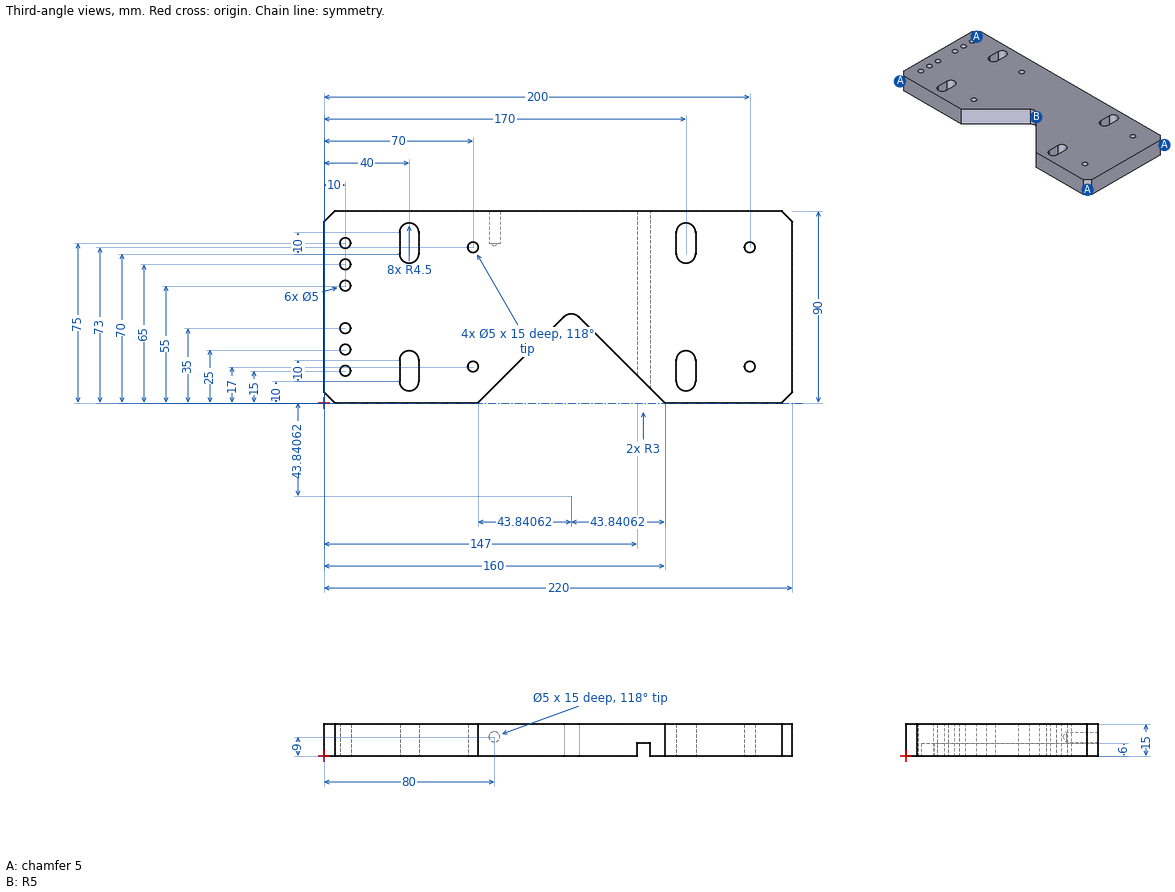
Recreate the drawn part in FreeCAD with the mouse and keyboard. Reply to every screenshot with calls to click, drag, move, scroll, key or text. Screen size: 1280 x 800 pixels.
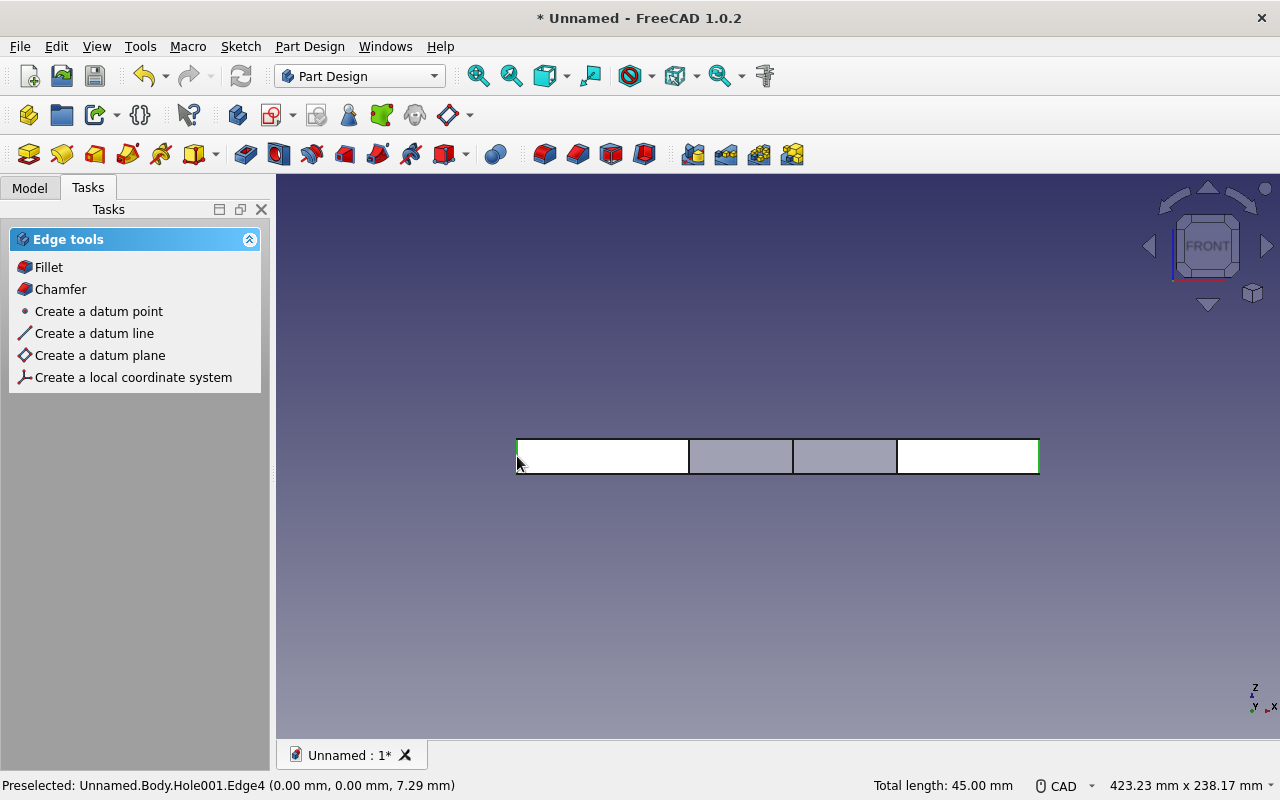
key(3)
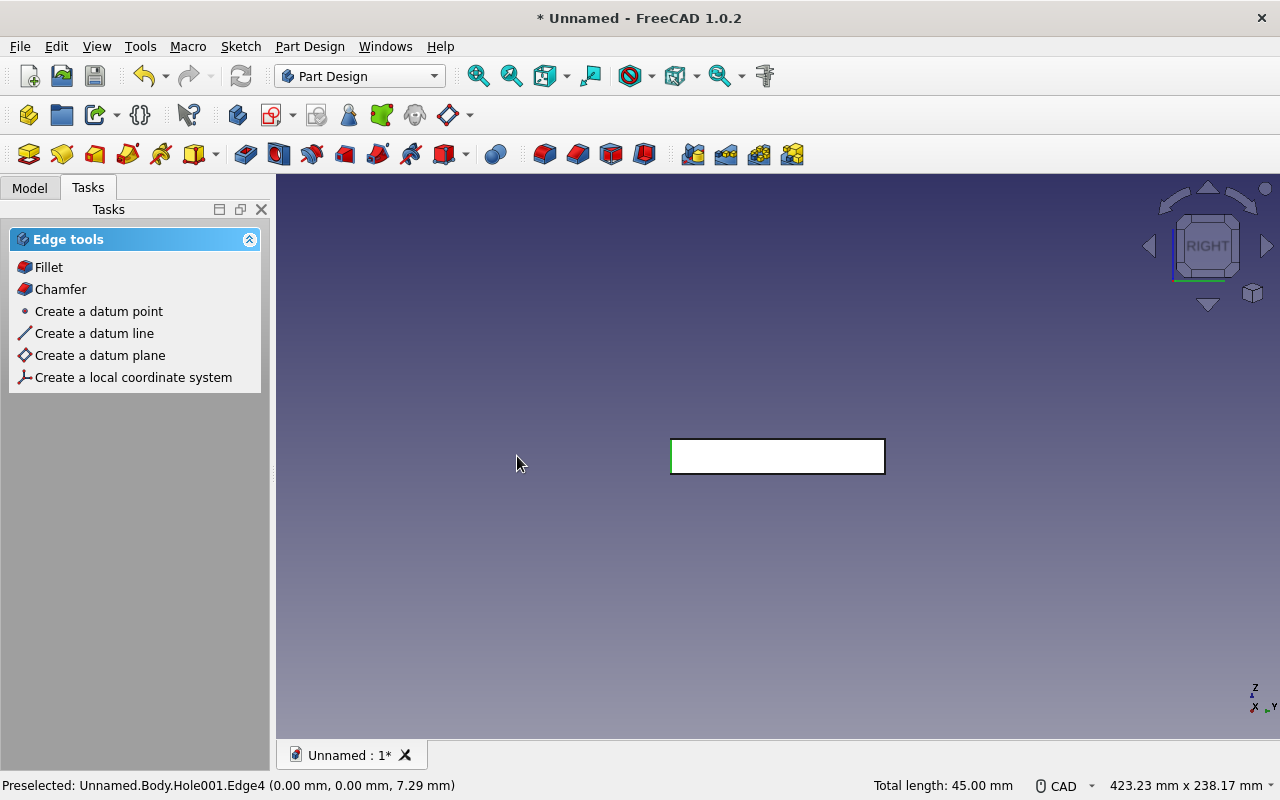
key(v)
key(f)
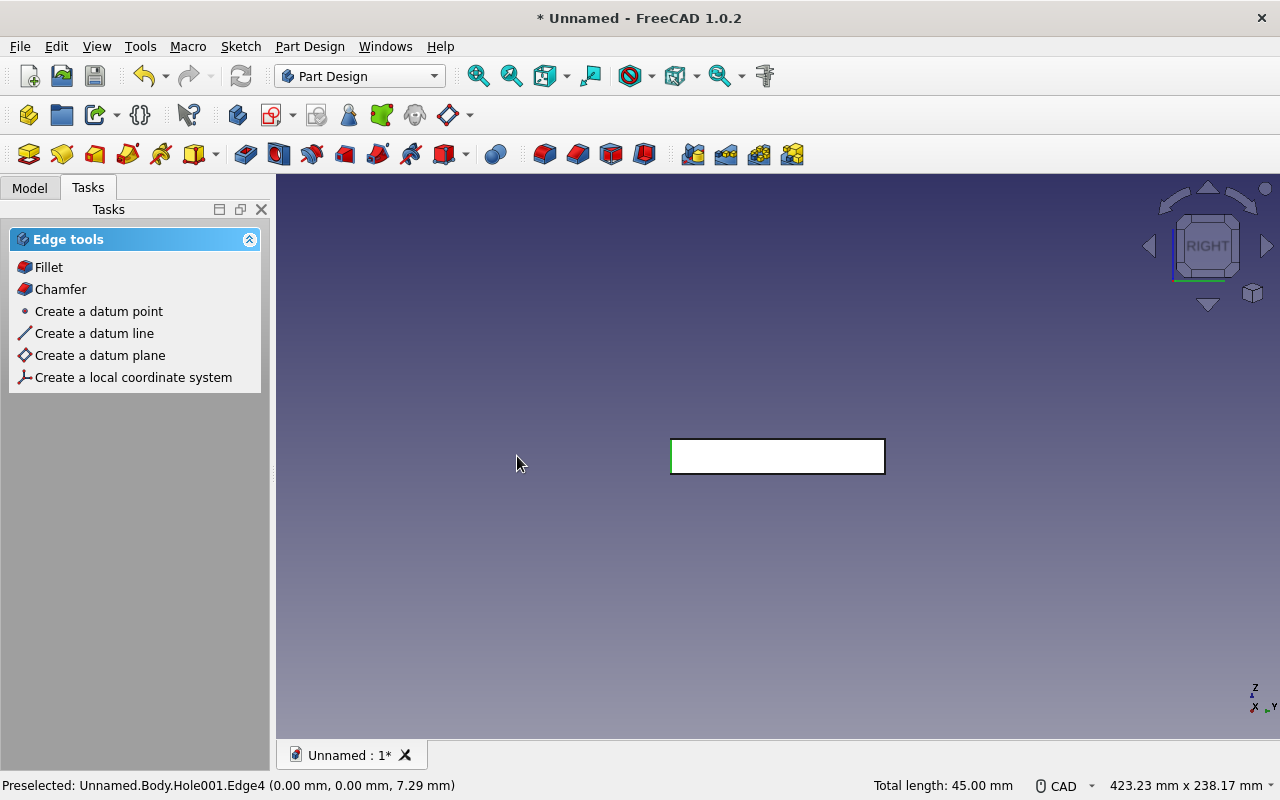
click(885, 455, ctrl)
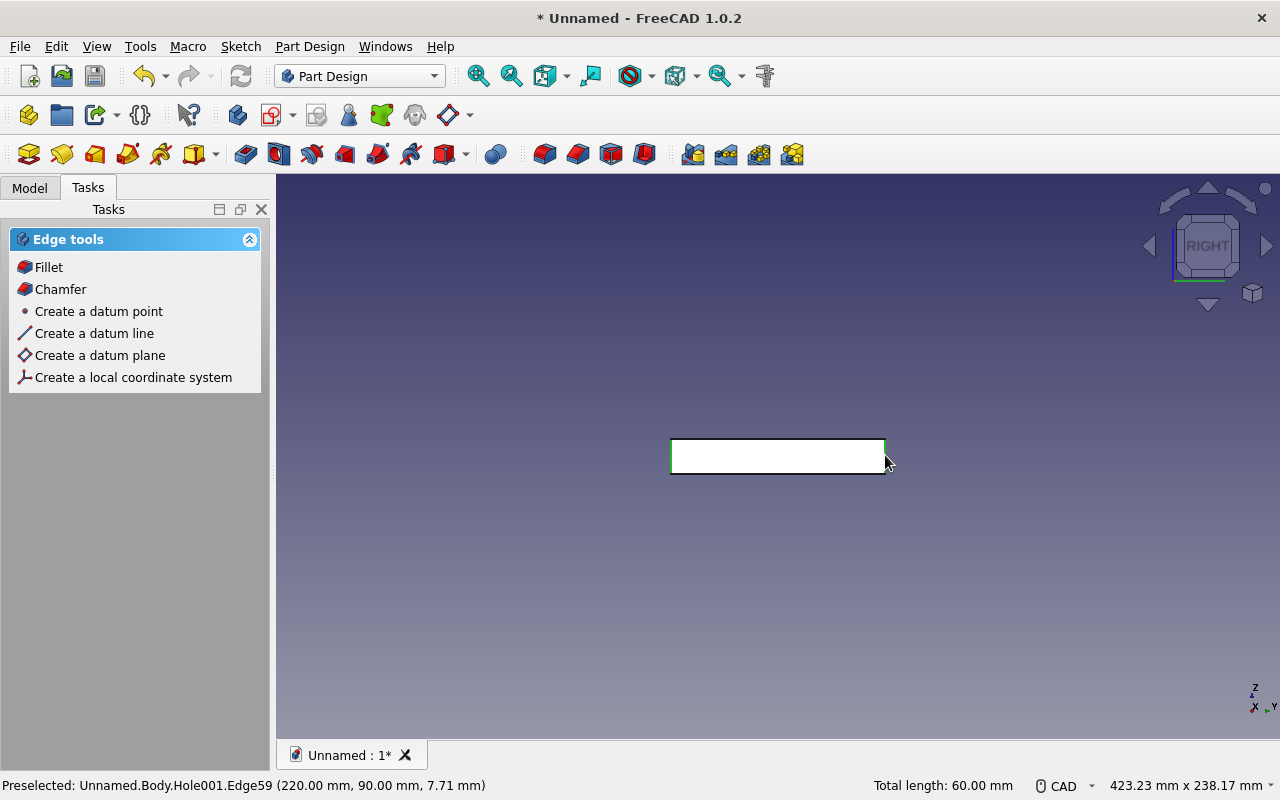
click(578, 154)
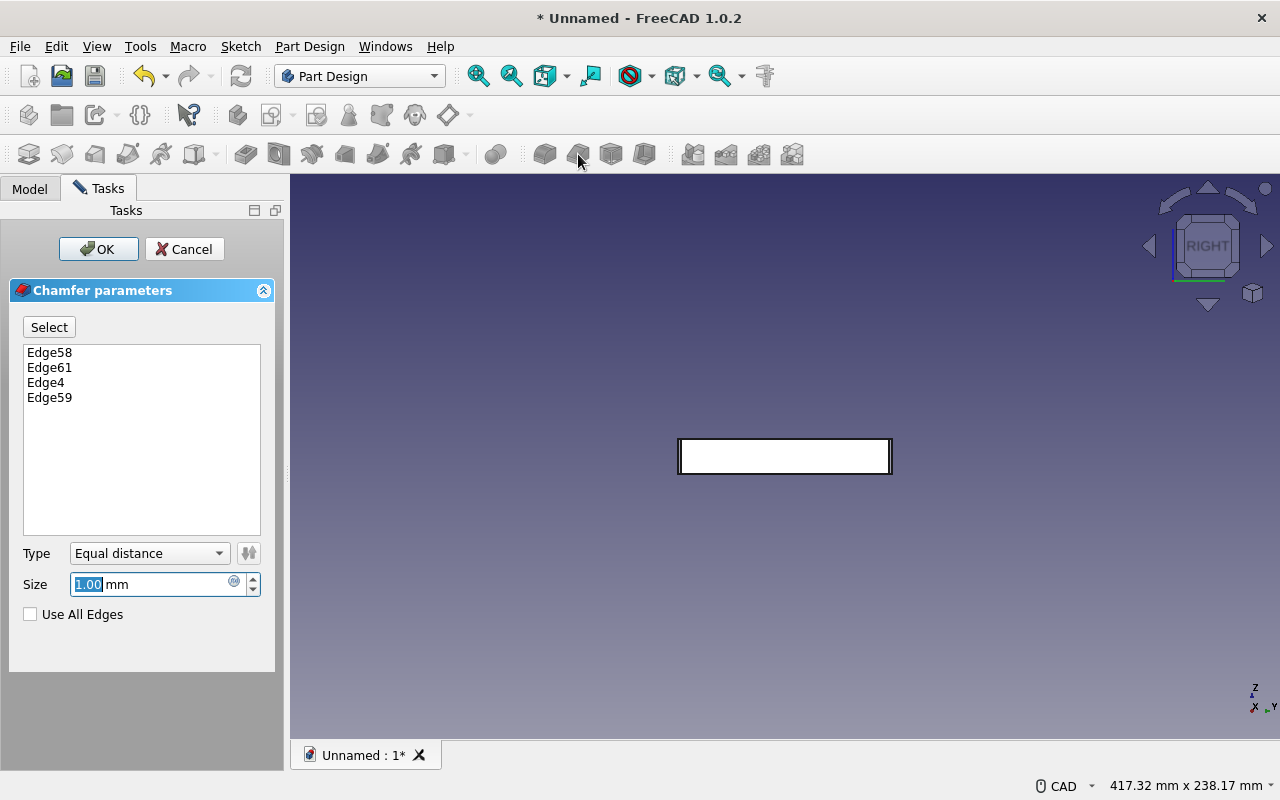
text(5)
key(Tab)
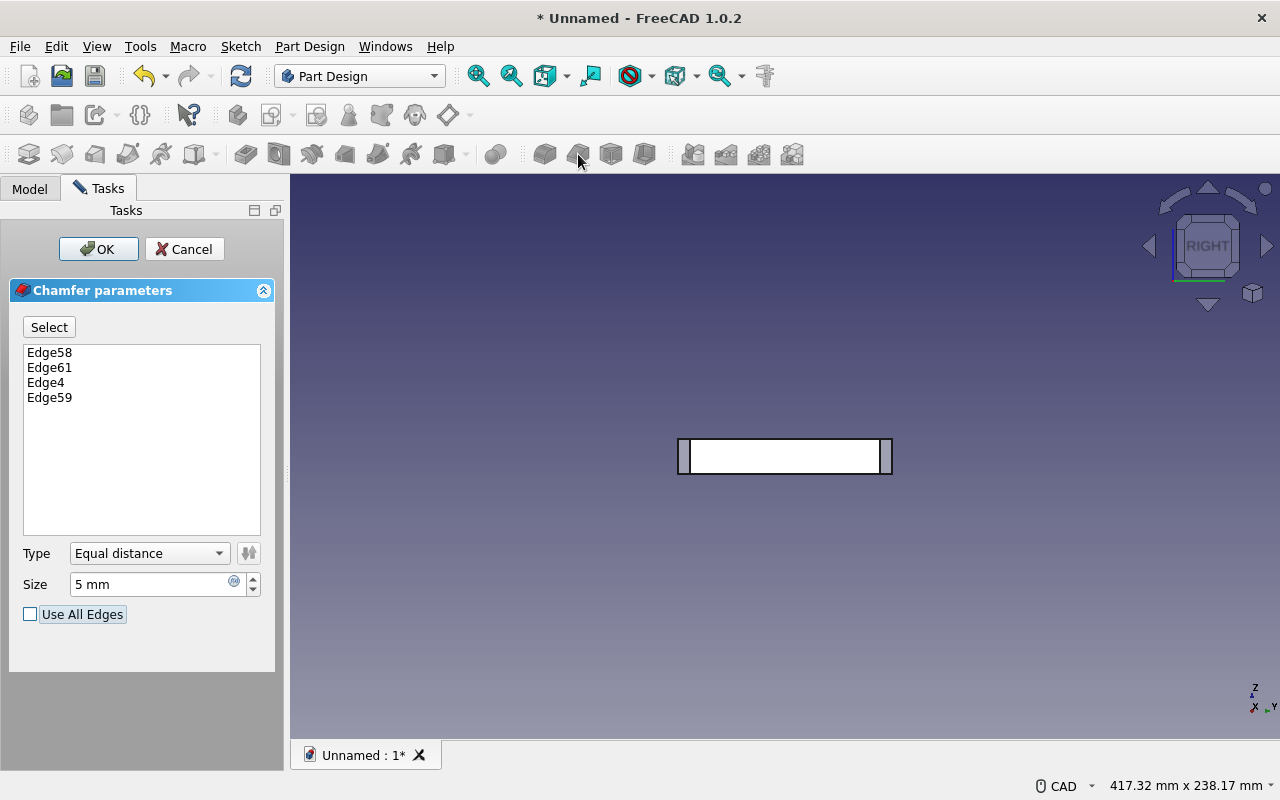
click(99, 249)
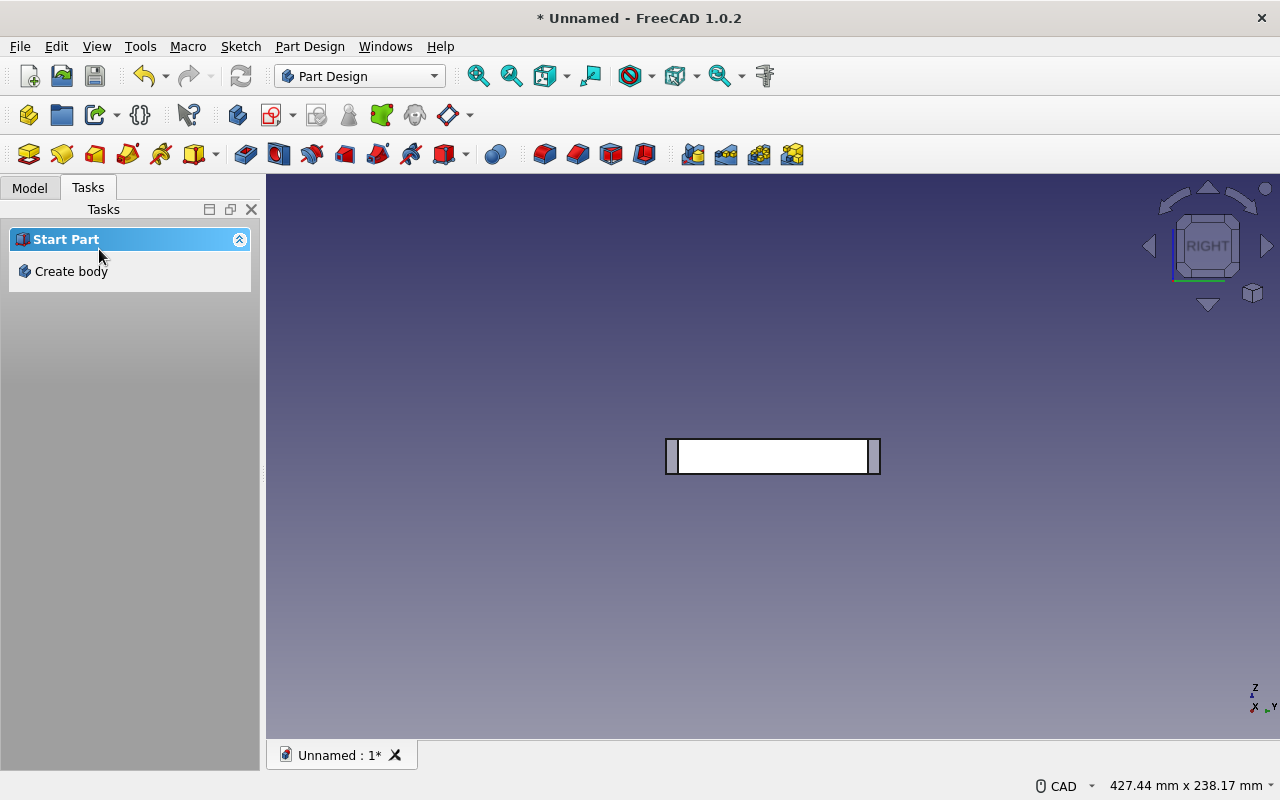
key(v)
key(f)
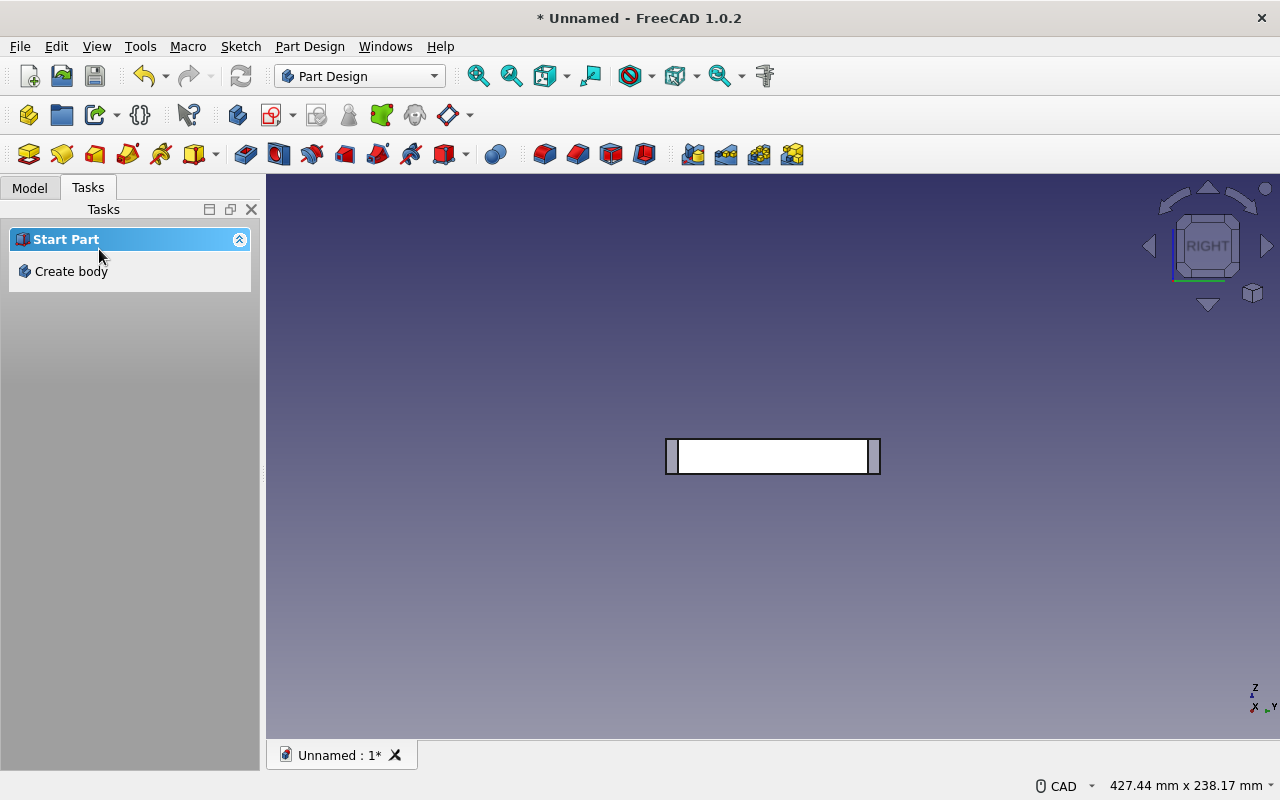
key(0)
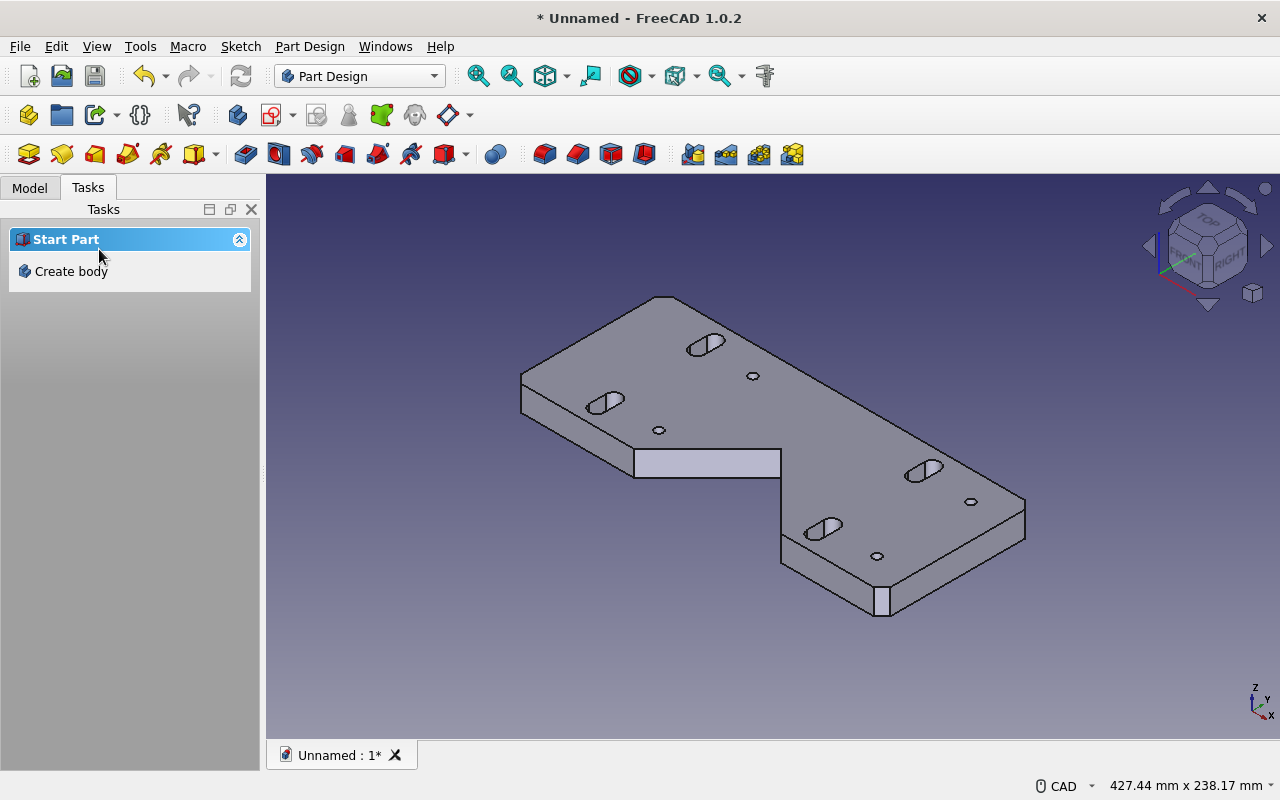
key(2)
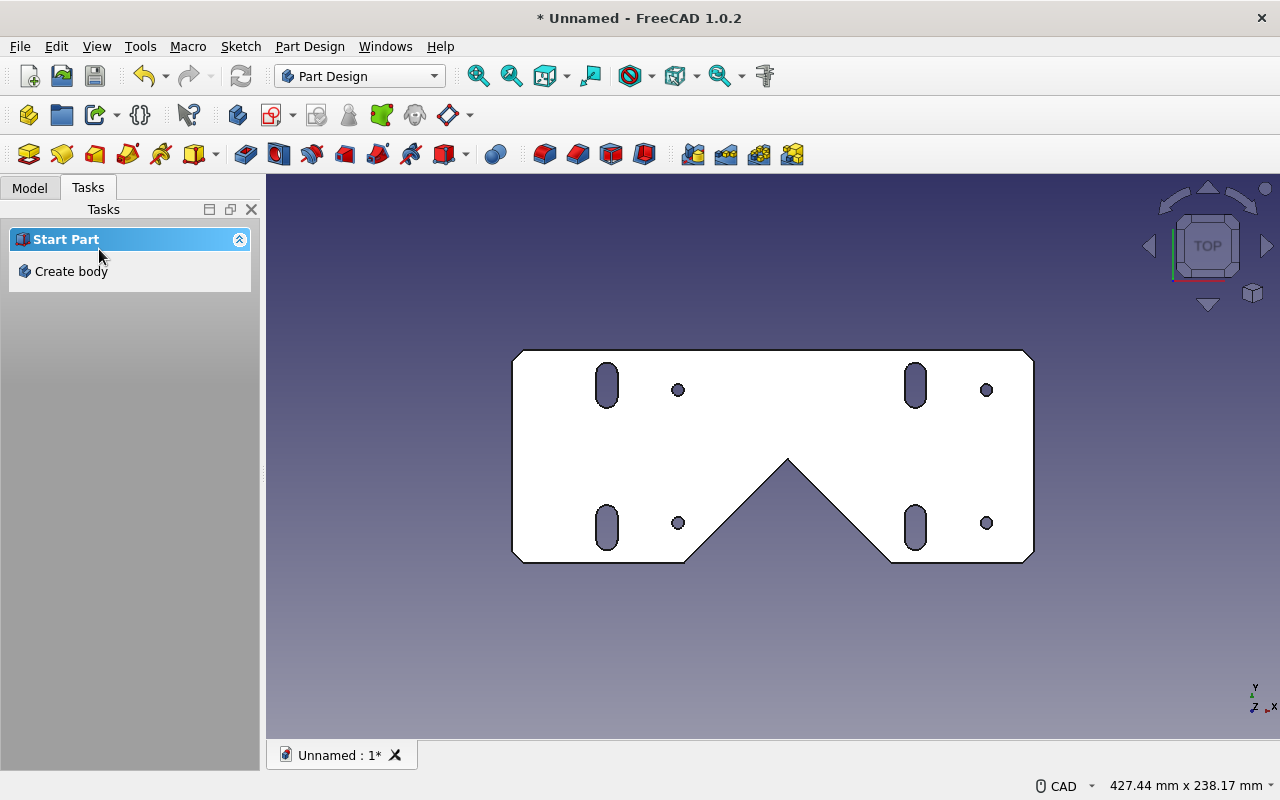
key(1)